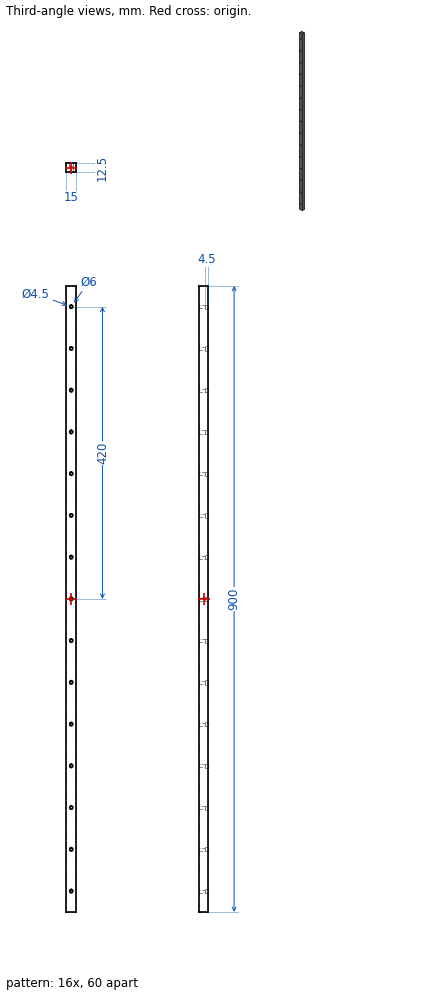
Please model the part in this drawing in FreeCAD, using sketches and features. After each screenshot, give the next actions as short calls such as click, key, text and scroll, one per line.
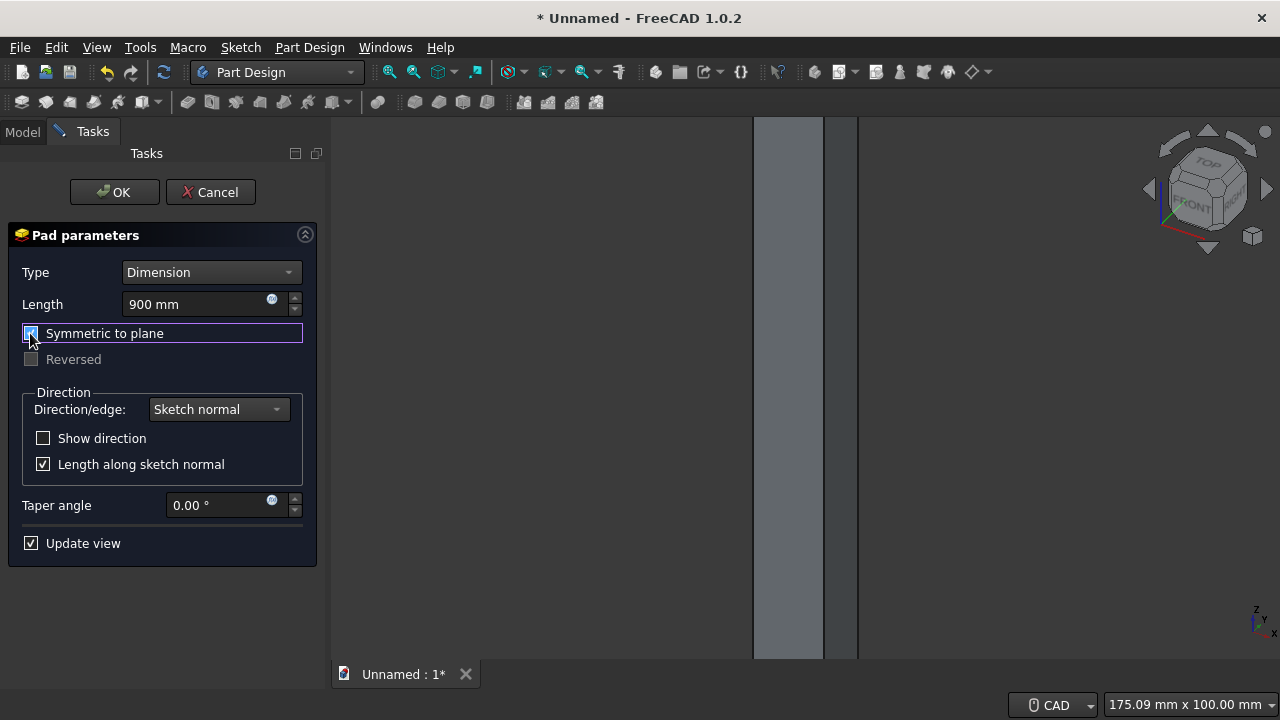
click(115, 192)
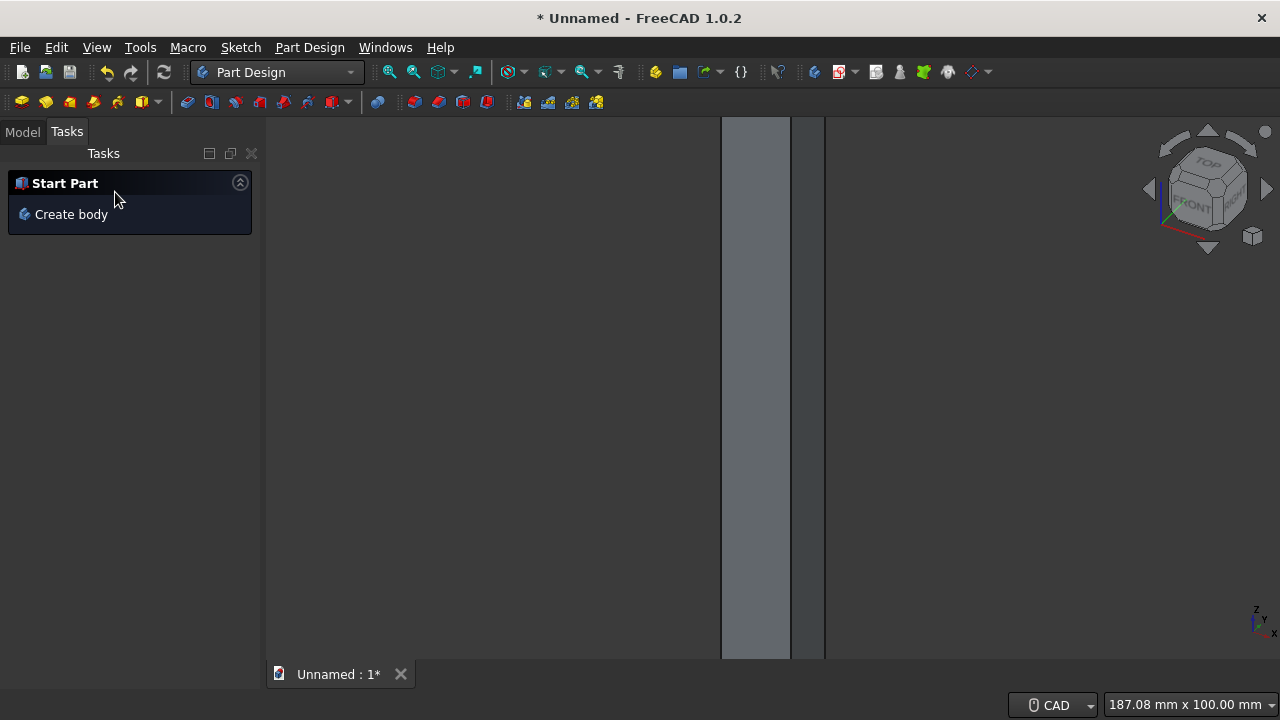
click(390, 72)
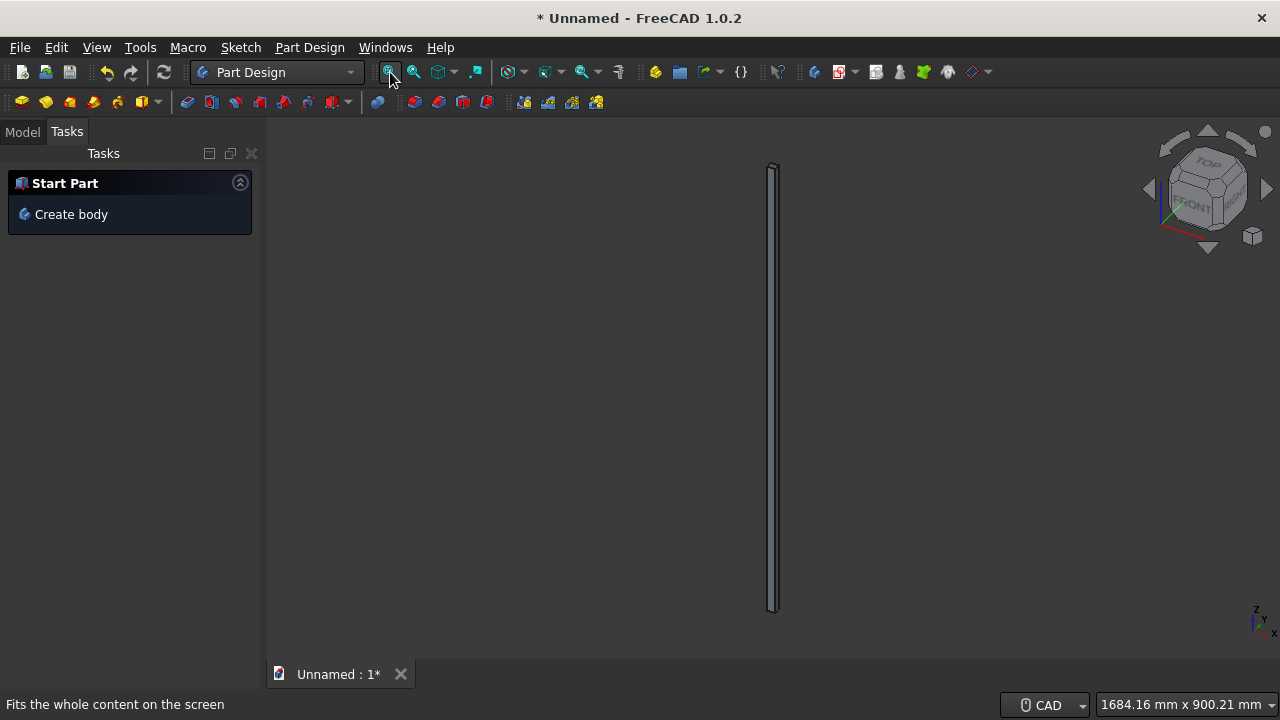
key(4)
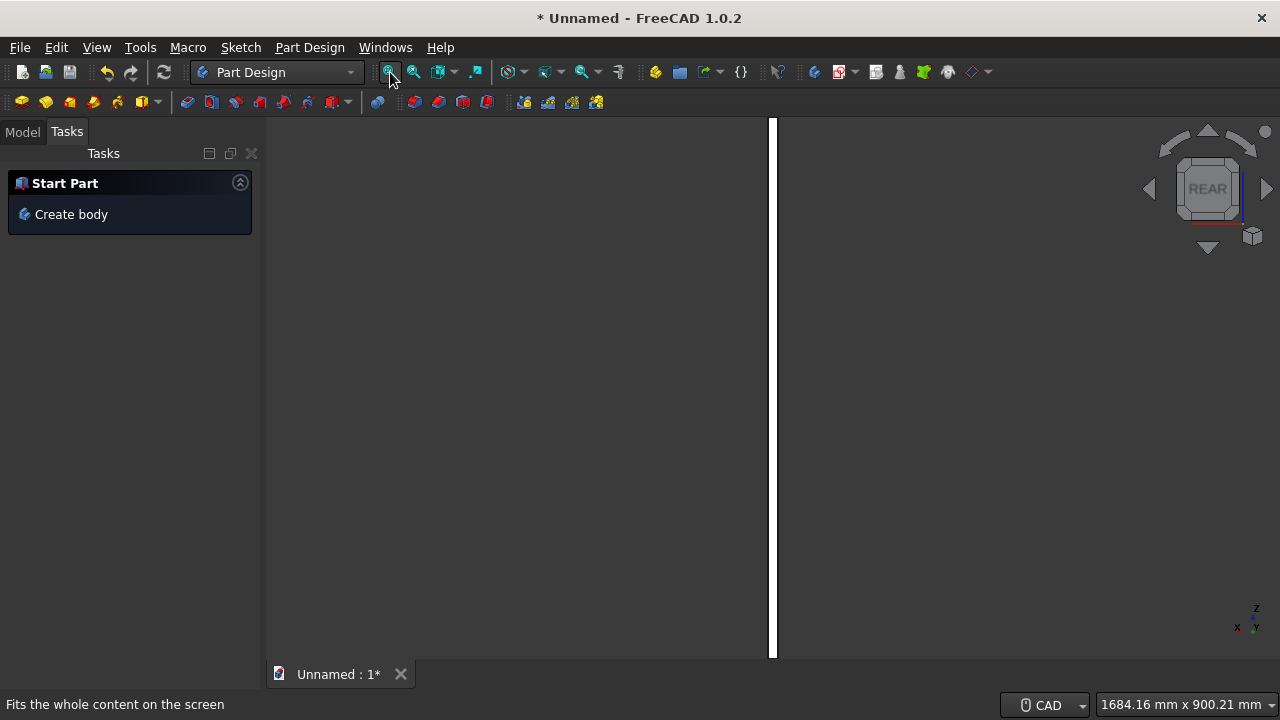
click(390, 72)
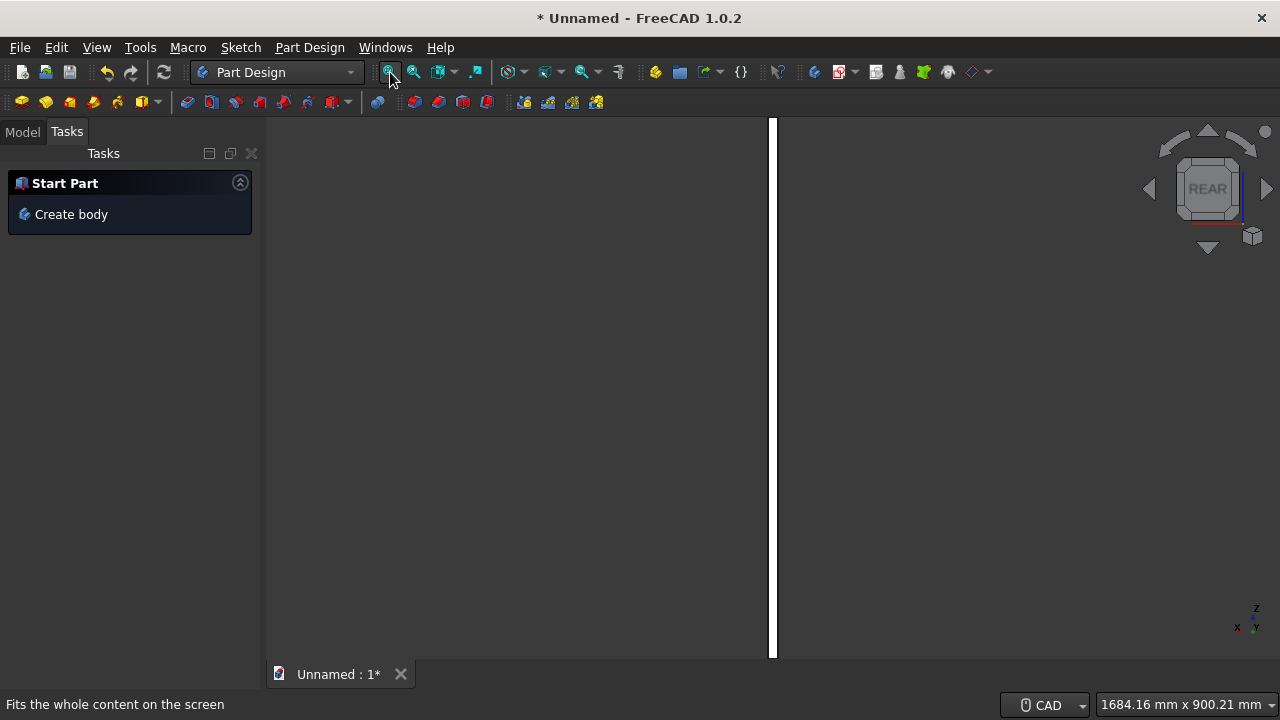
scroll(773, 155, up, 5)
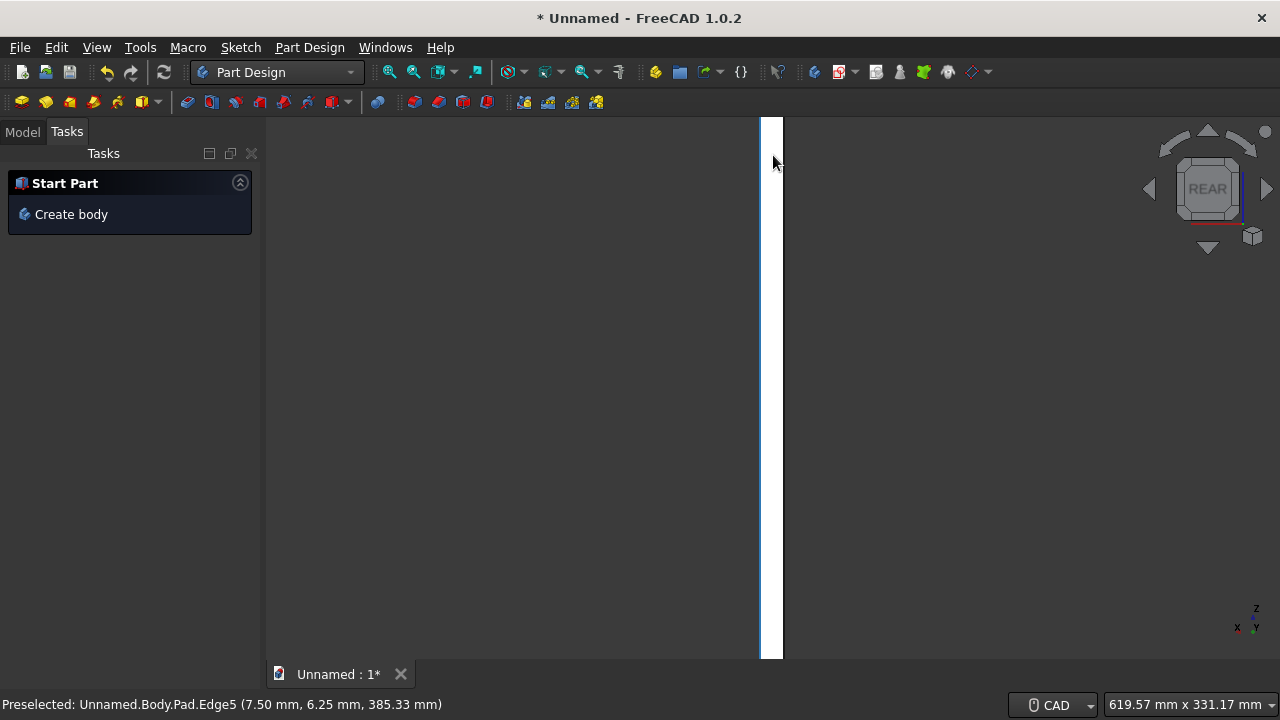
click(772, 156)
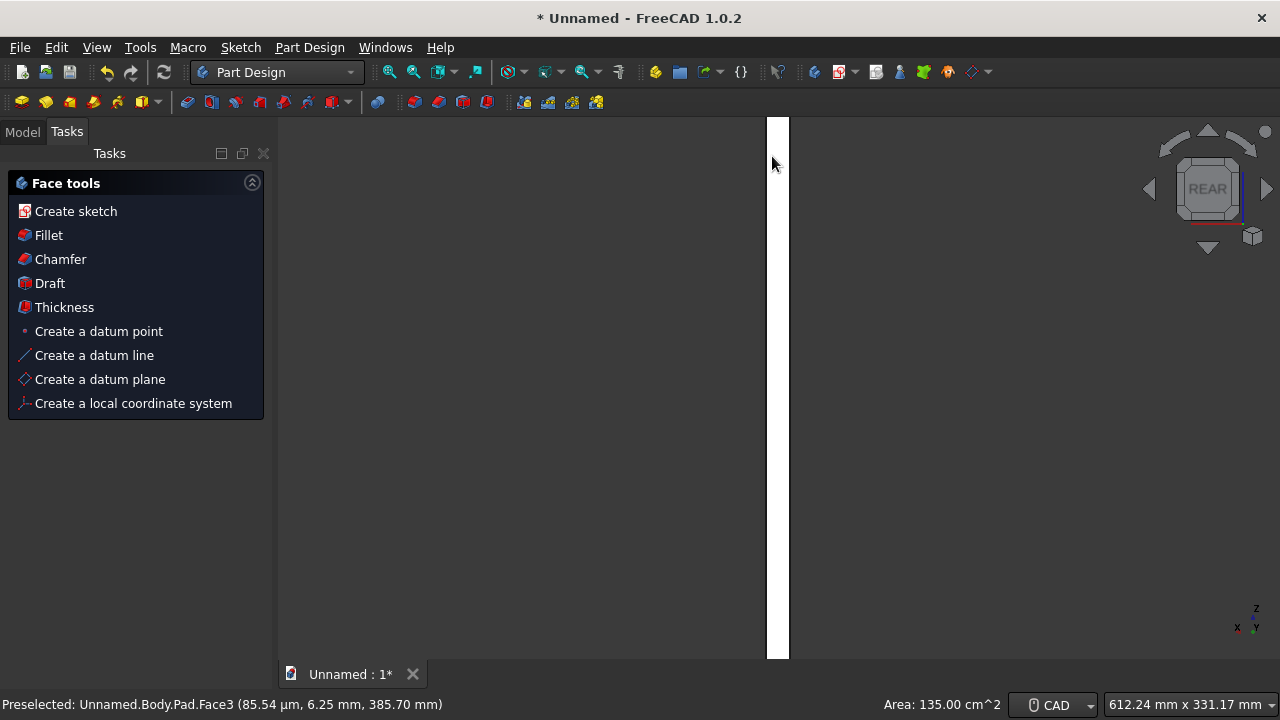
click(840, 72)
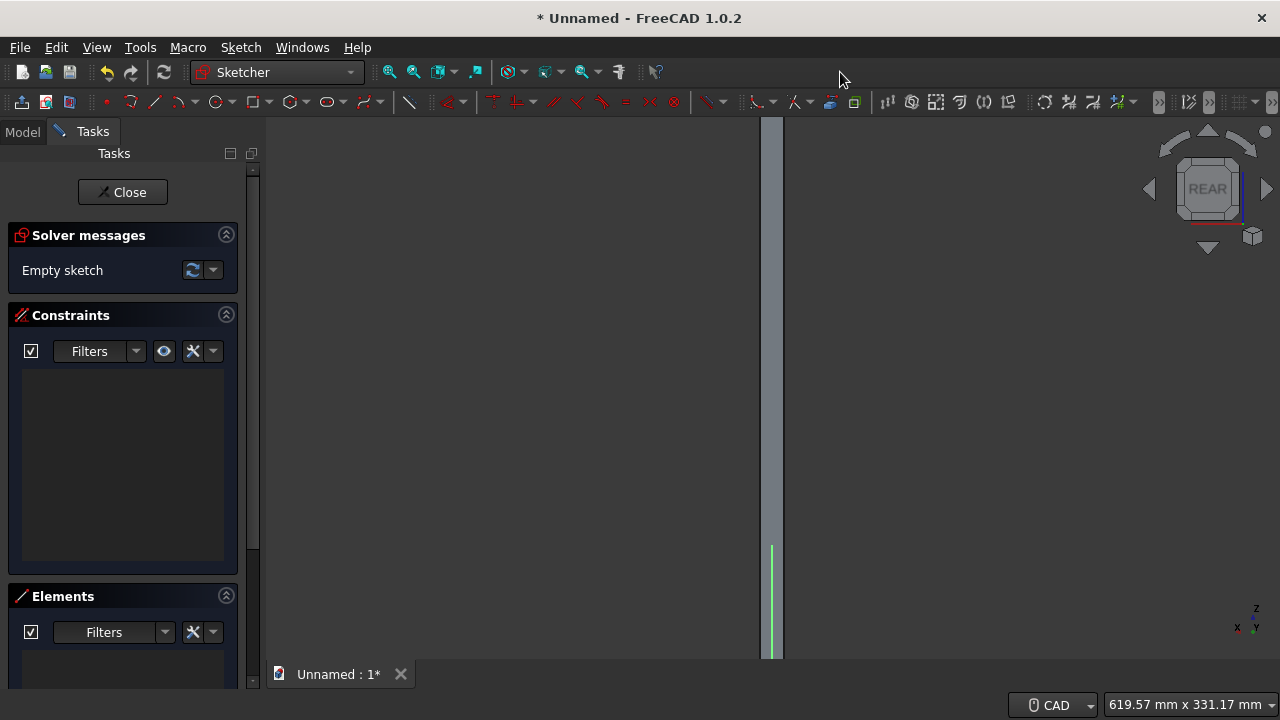
scroll(704, 388, down, 5)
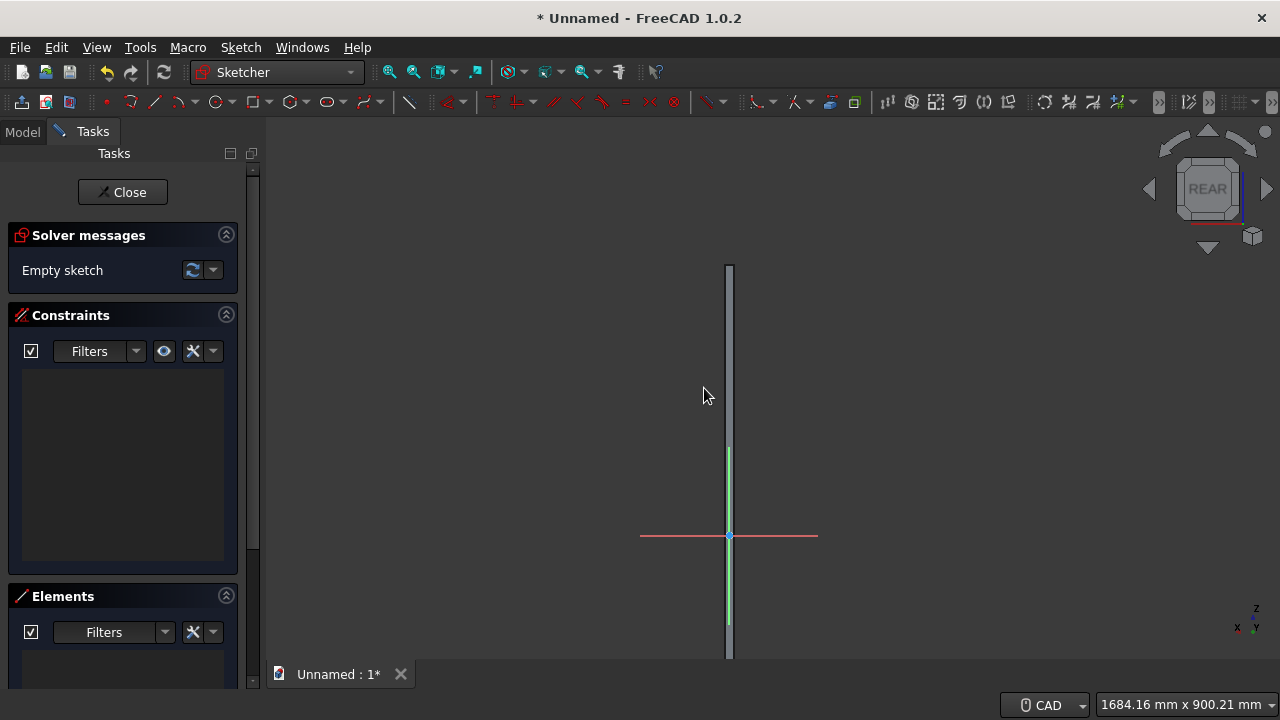
scroll(731, 277, up, 15)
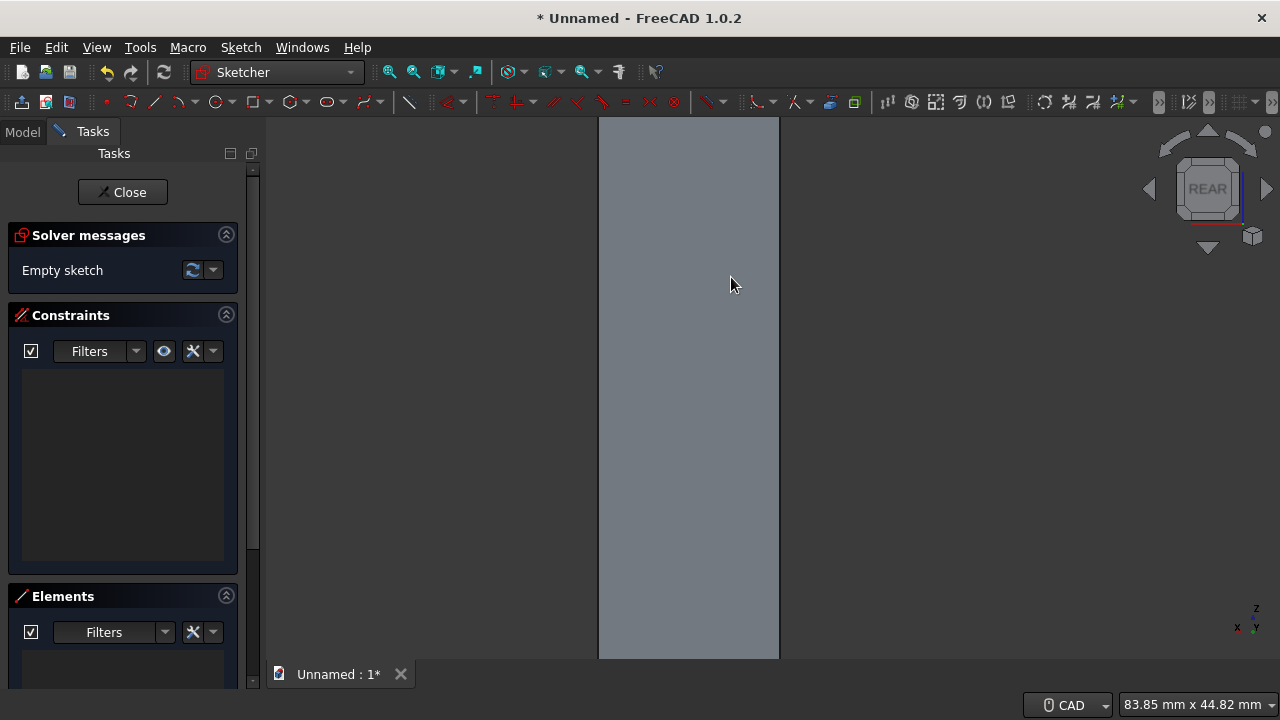
scroll(685, 385, up, 8)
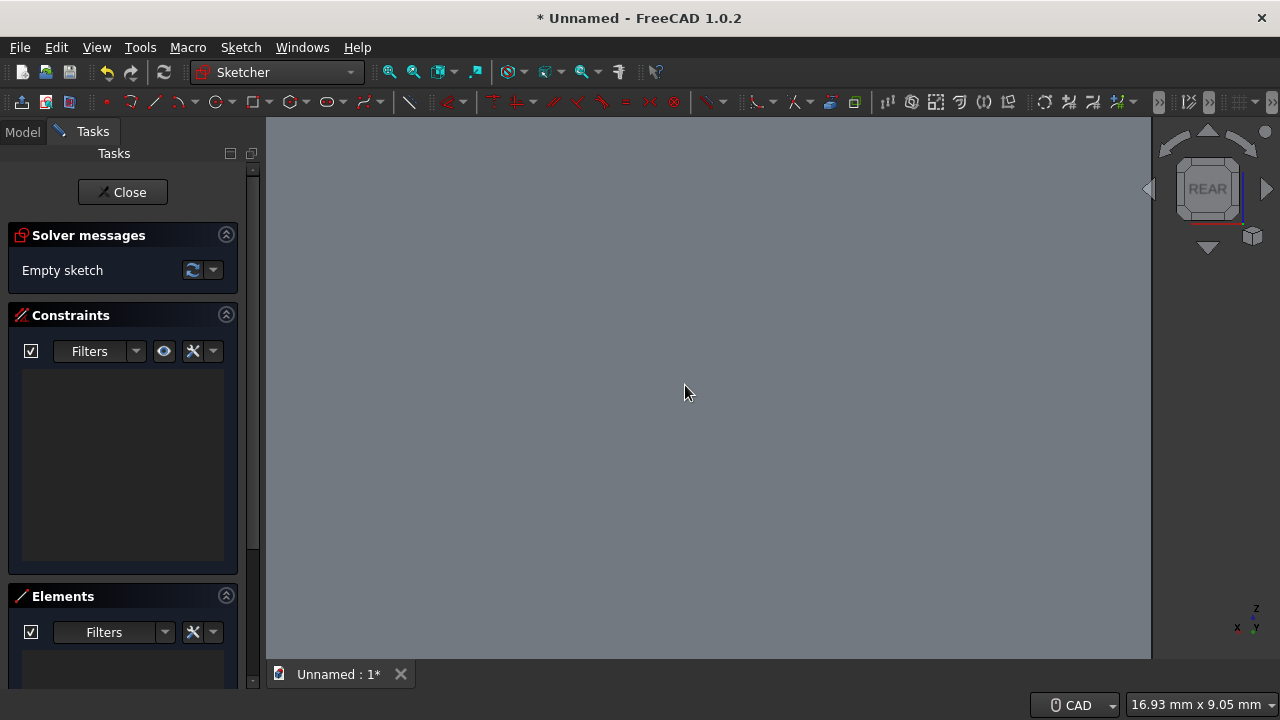
click(216, 102)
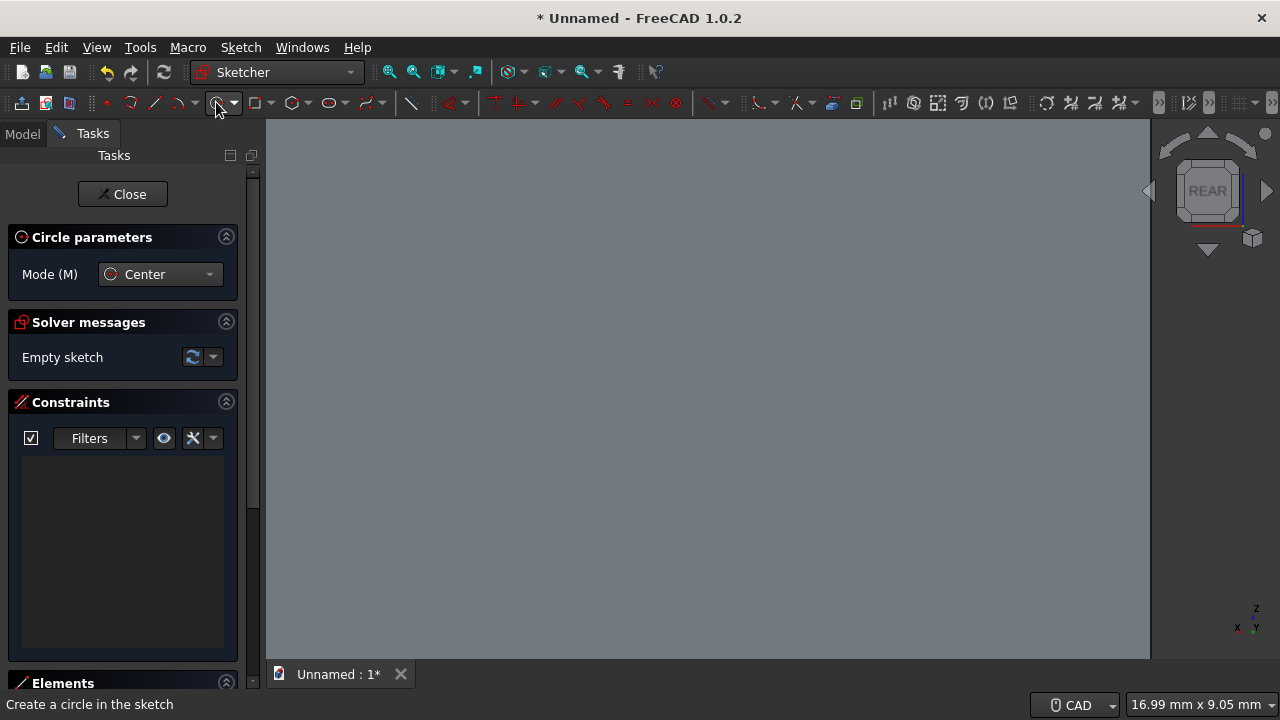
click(703, 386)
move(830, 260)